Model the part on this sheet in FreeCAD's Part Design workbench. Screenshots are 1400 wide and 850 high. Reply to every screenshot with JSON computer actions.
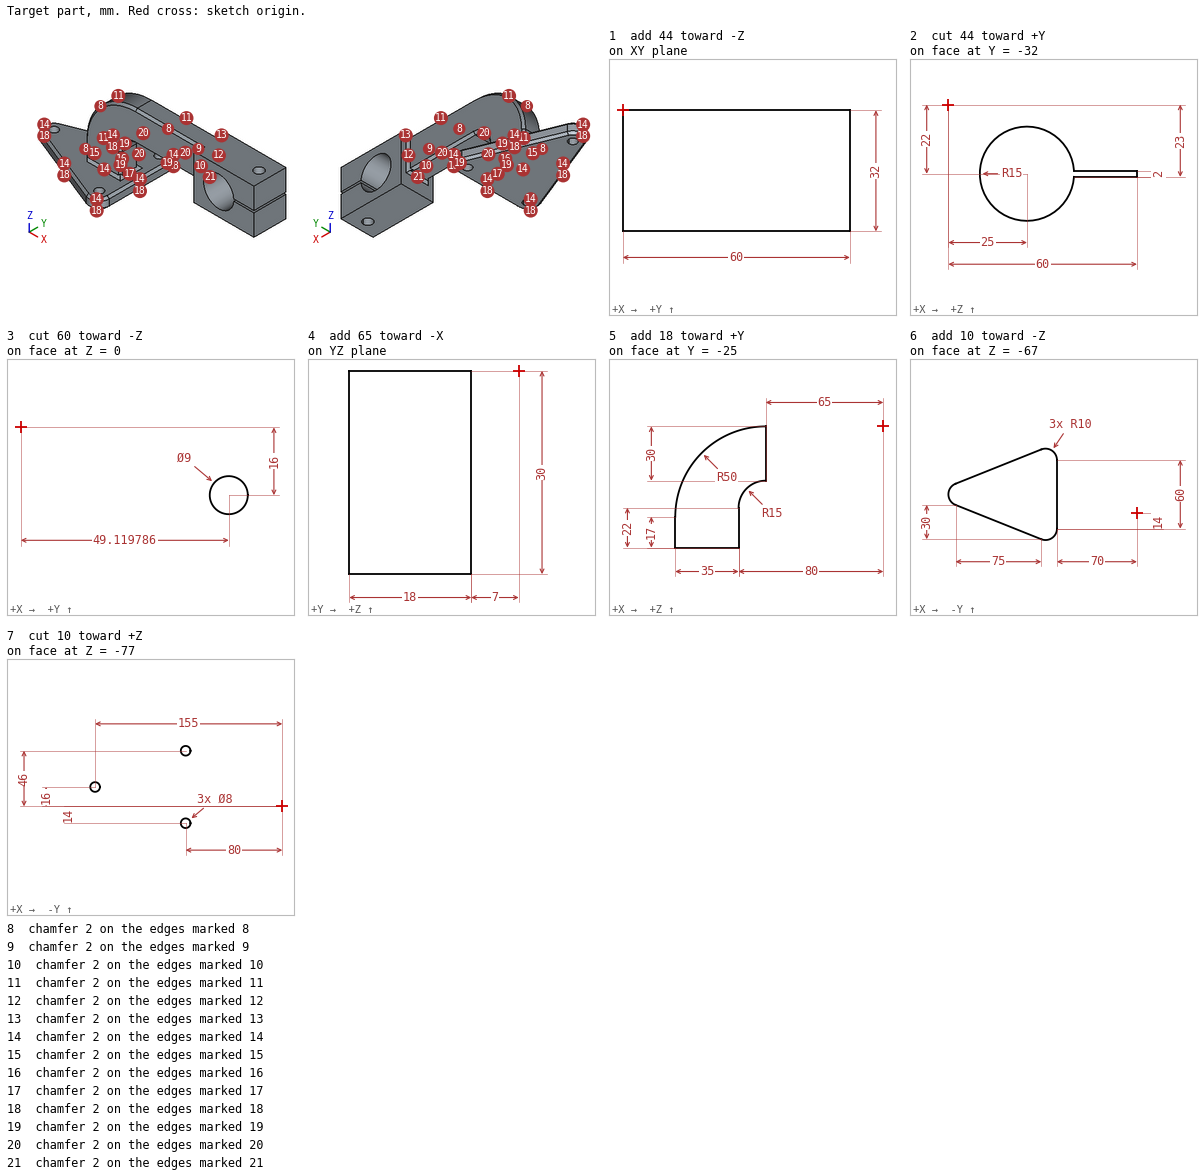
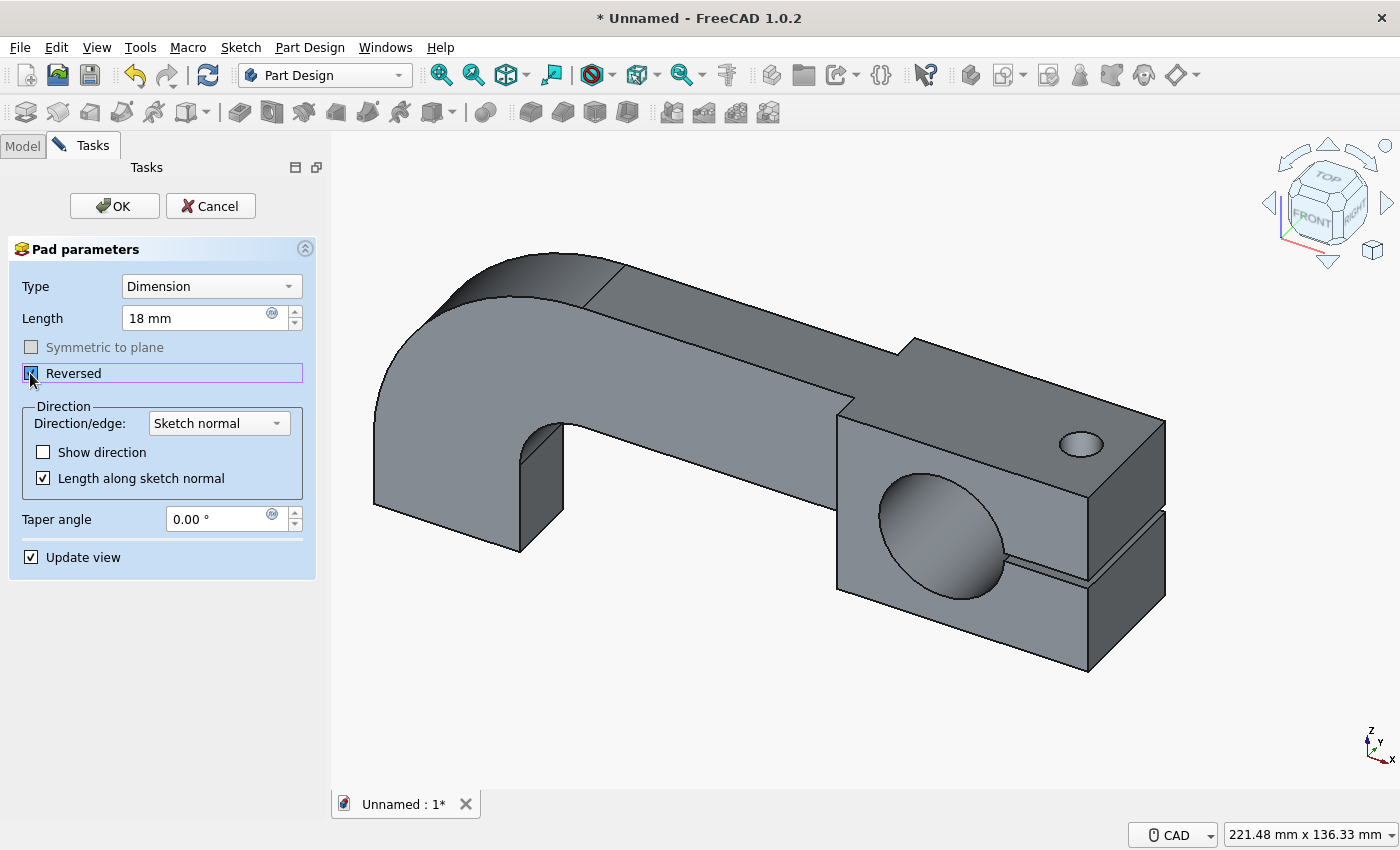
{"action": "left_click", "coordinate": [115, 206]}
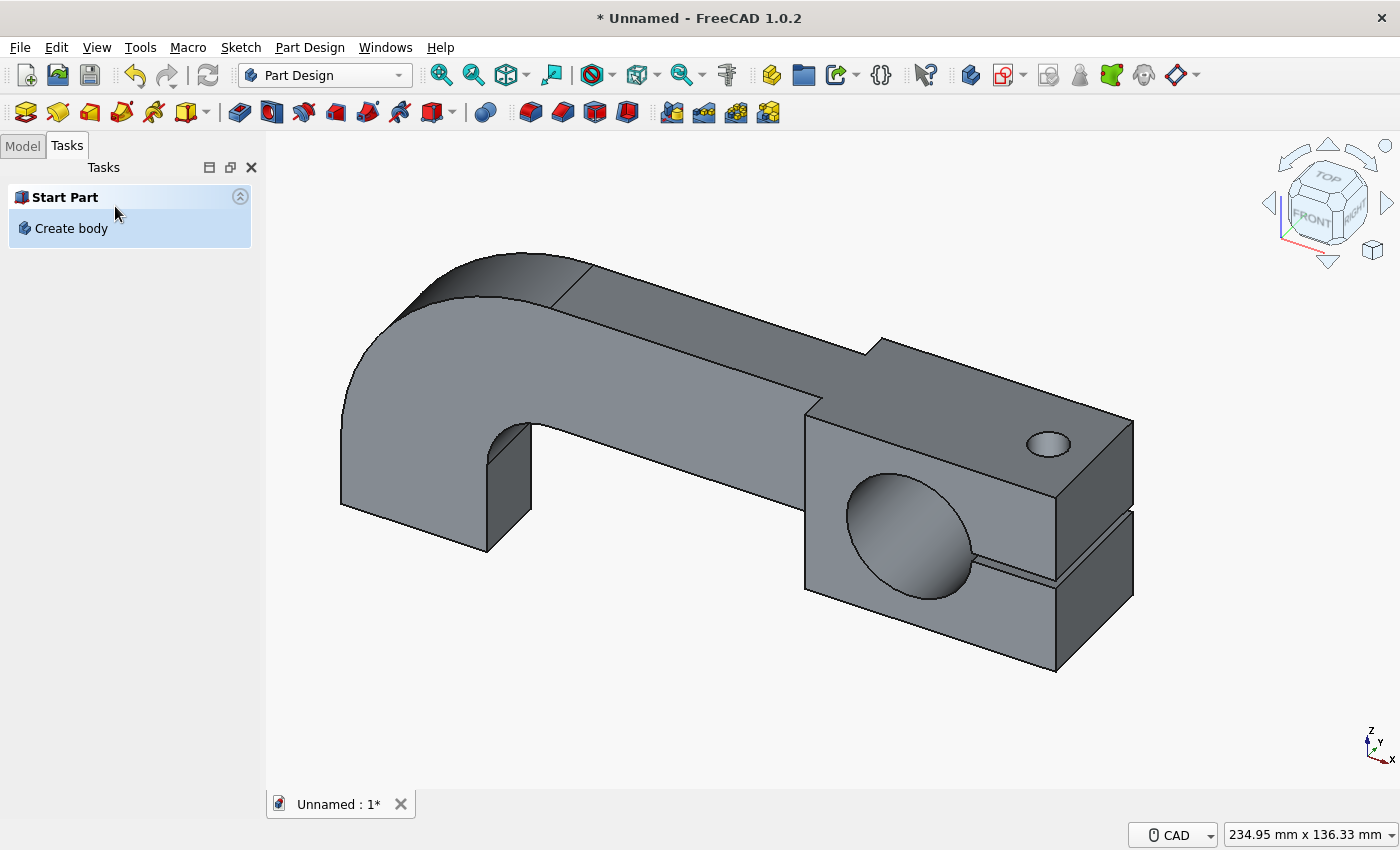
{"action": "key", "text": "5"}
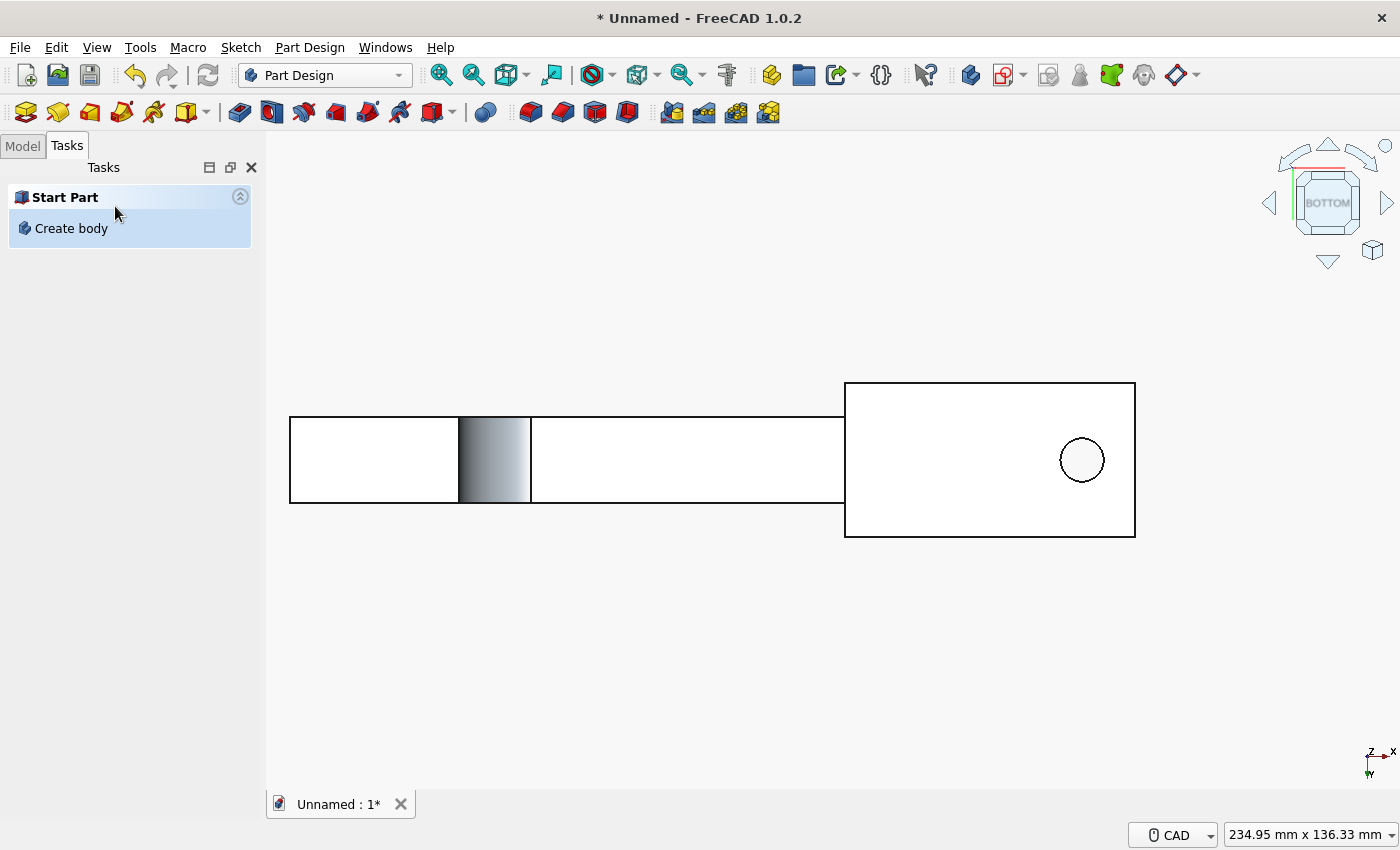
{"action": "left_click", "coordinate": [399, 459]}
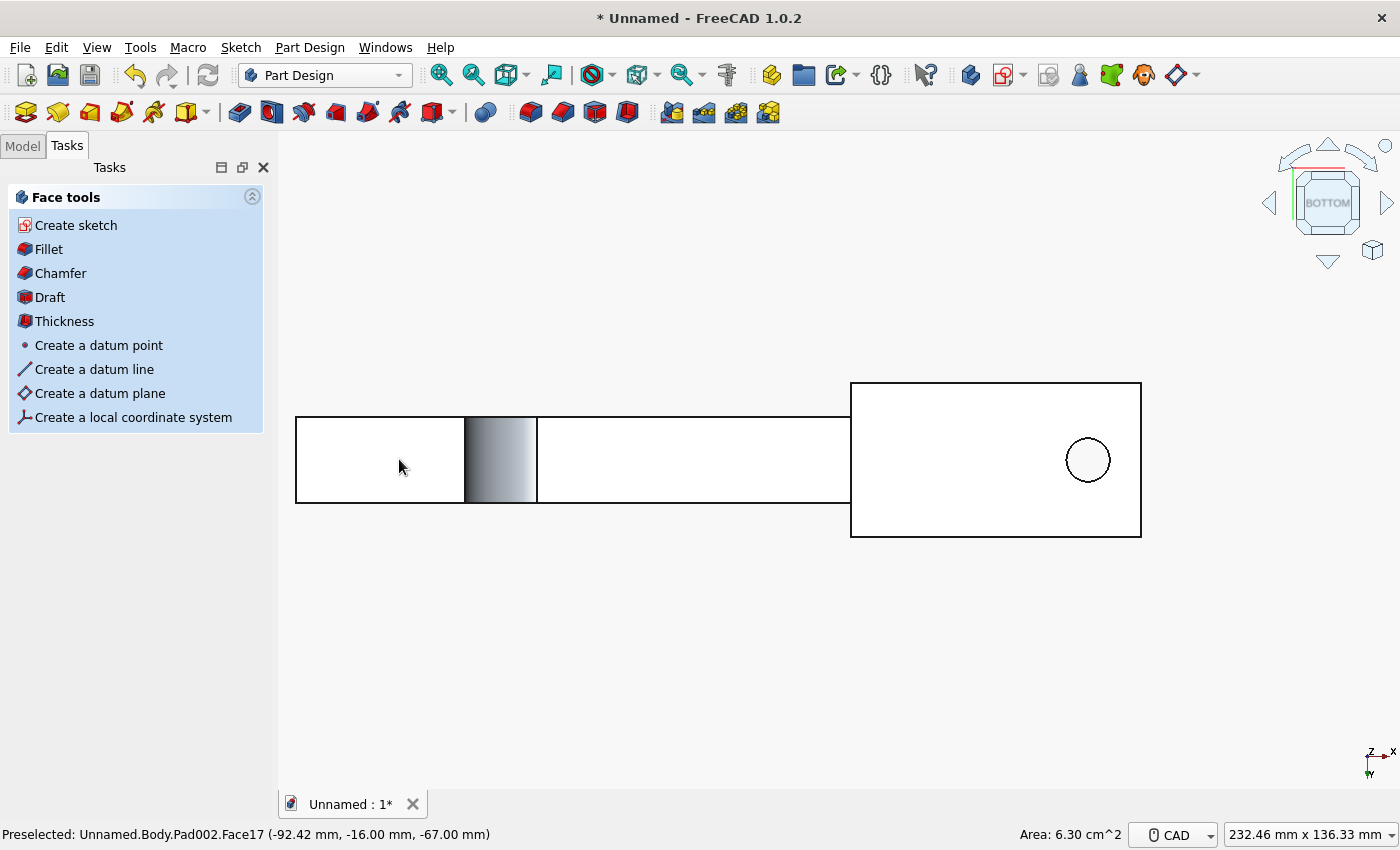
{"action": "left_click", "coordinate": [1004, 76]}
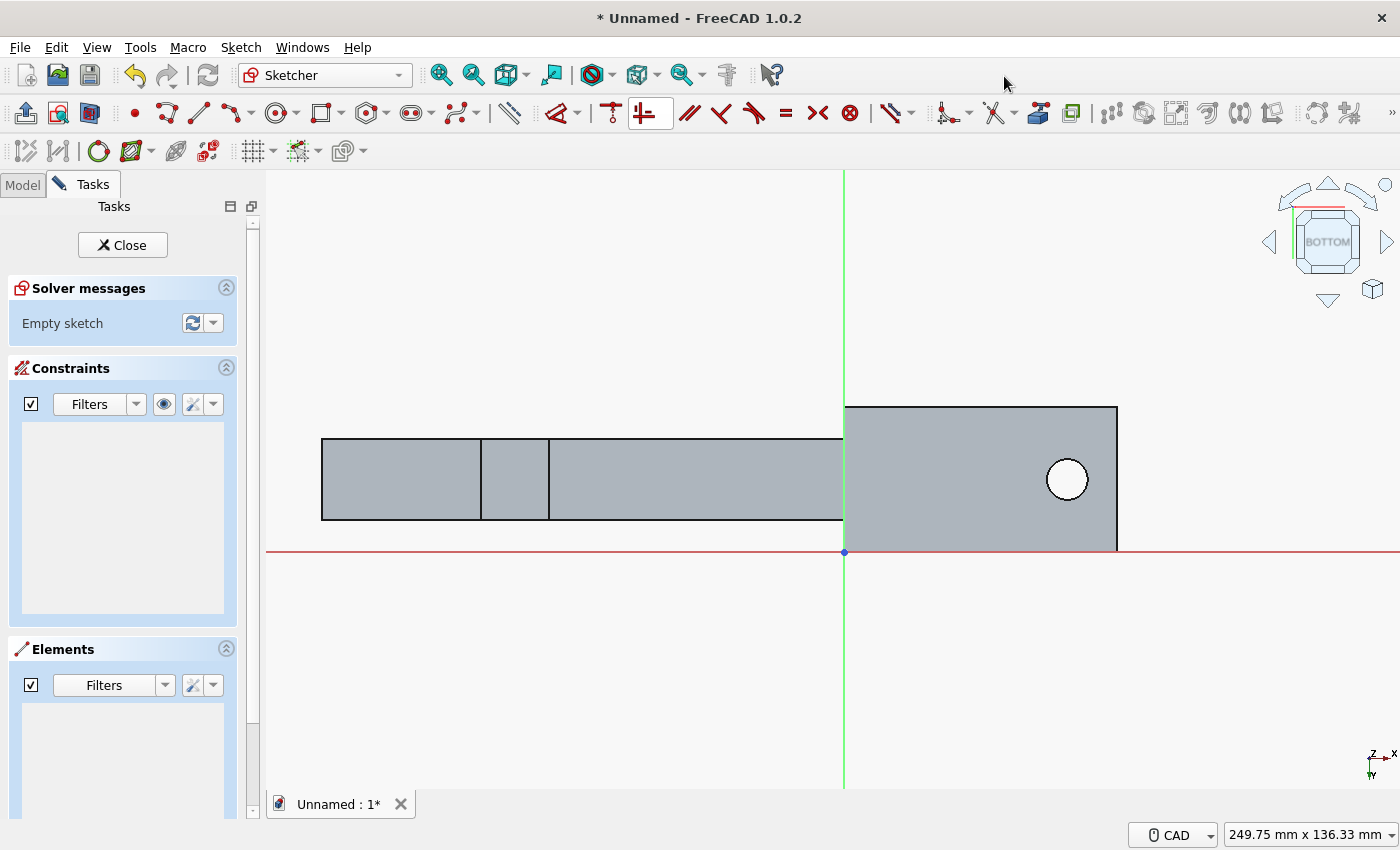
{"action": "scroll", "coordinate": [1235, 479], "scroll_direction": "down", "scroll_amount": 2}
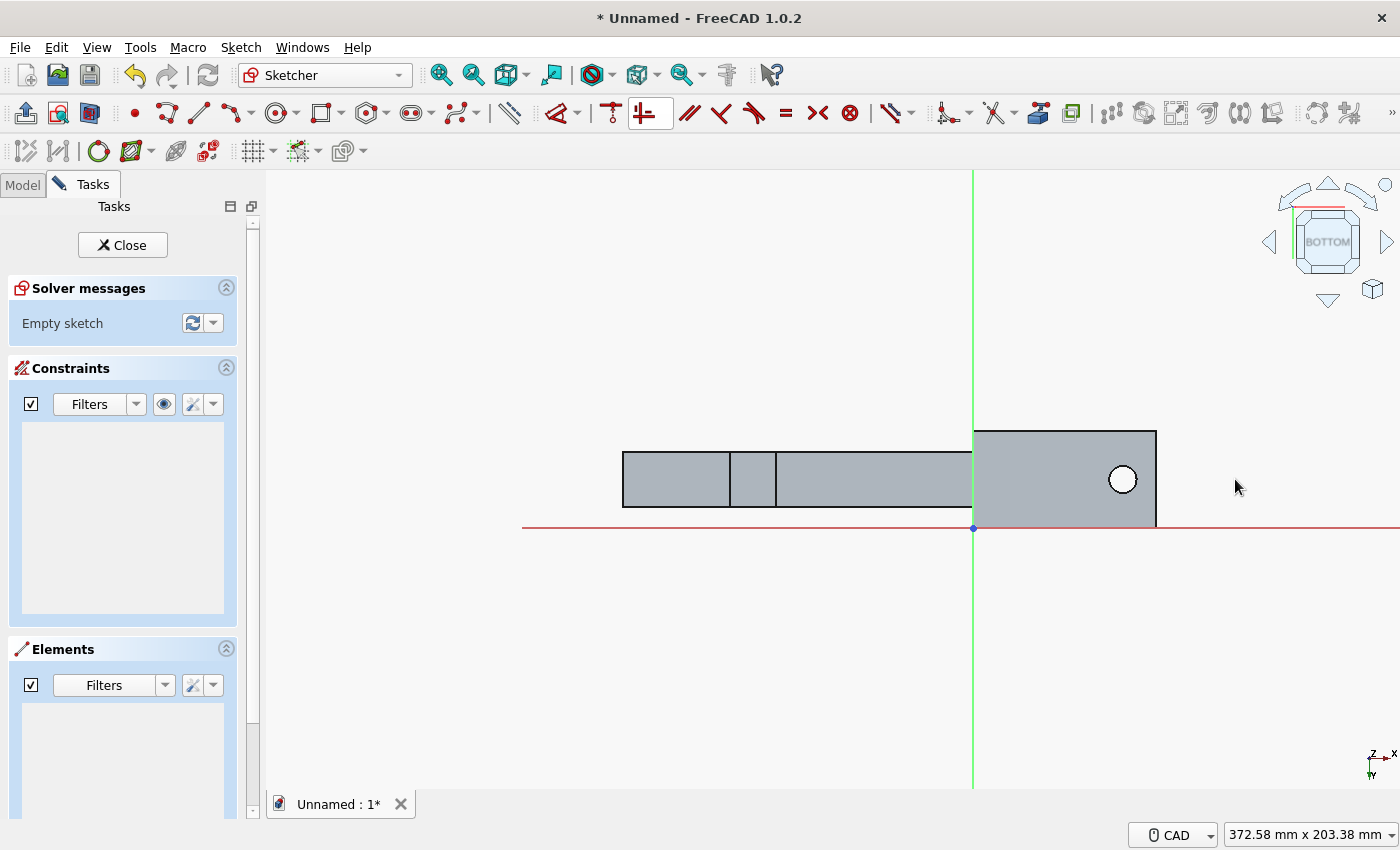
{"action": "left_click", "coordinate": [200, 114]}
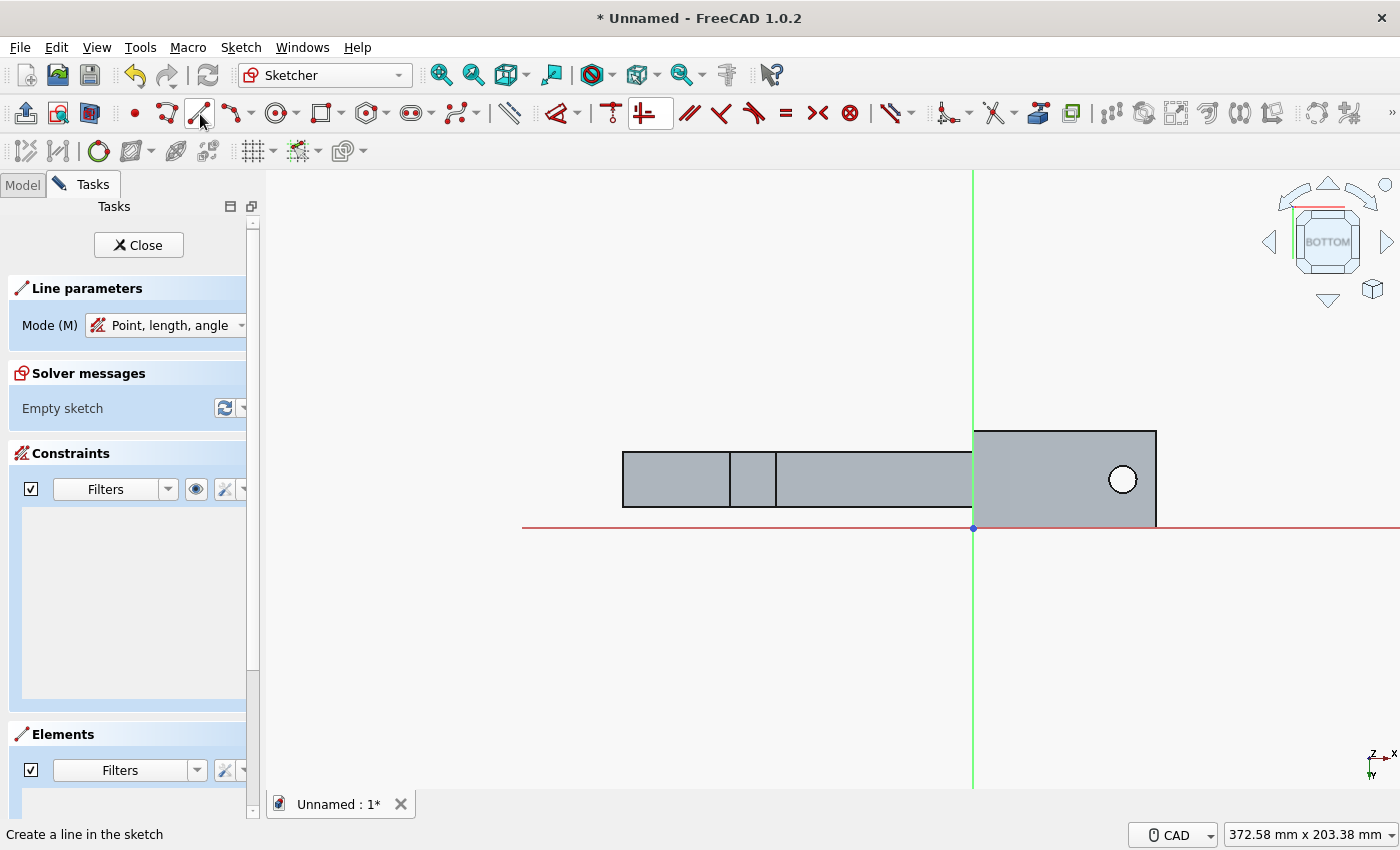
{"action": "left_click", "coordinate": [490, 508]}
{"action": "left_click", "coordinate": [719, 599]}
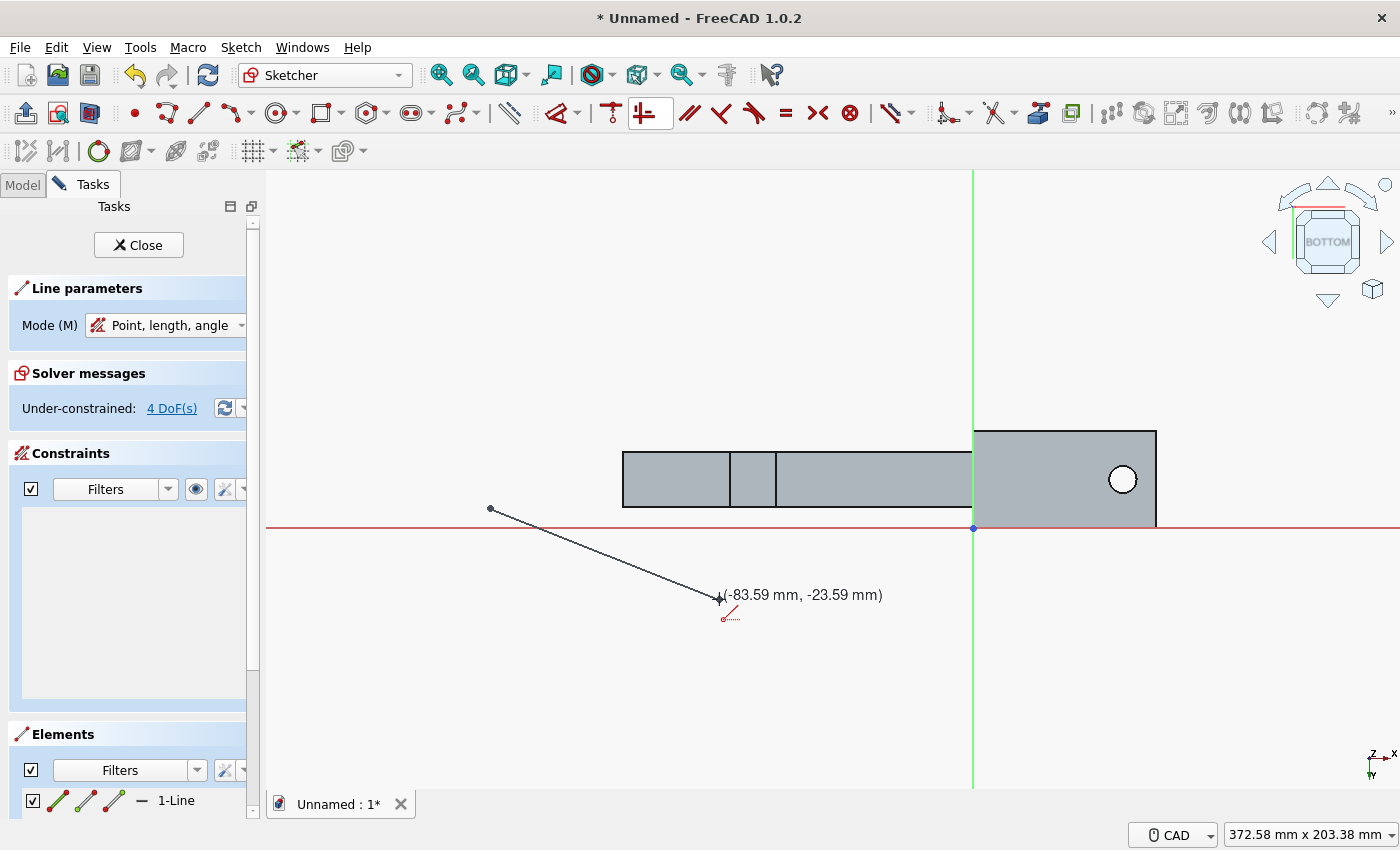
{"action": "left_click", "coordinate": [760, 571]}
{"action": "left_click", "coordinate": [760, 388]}